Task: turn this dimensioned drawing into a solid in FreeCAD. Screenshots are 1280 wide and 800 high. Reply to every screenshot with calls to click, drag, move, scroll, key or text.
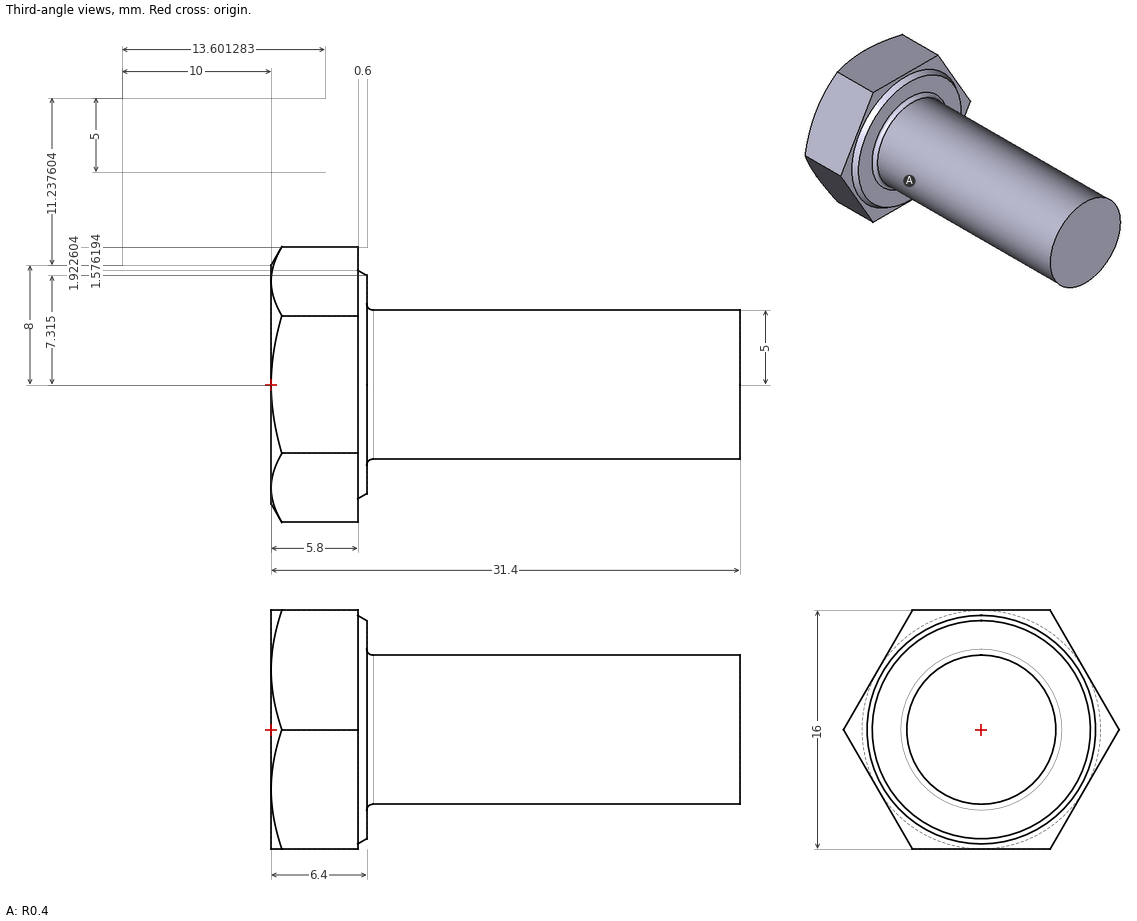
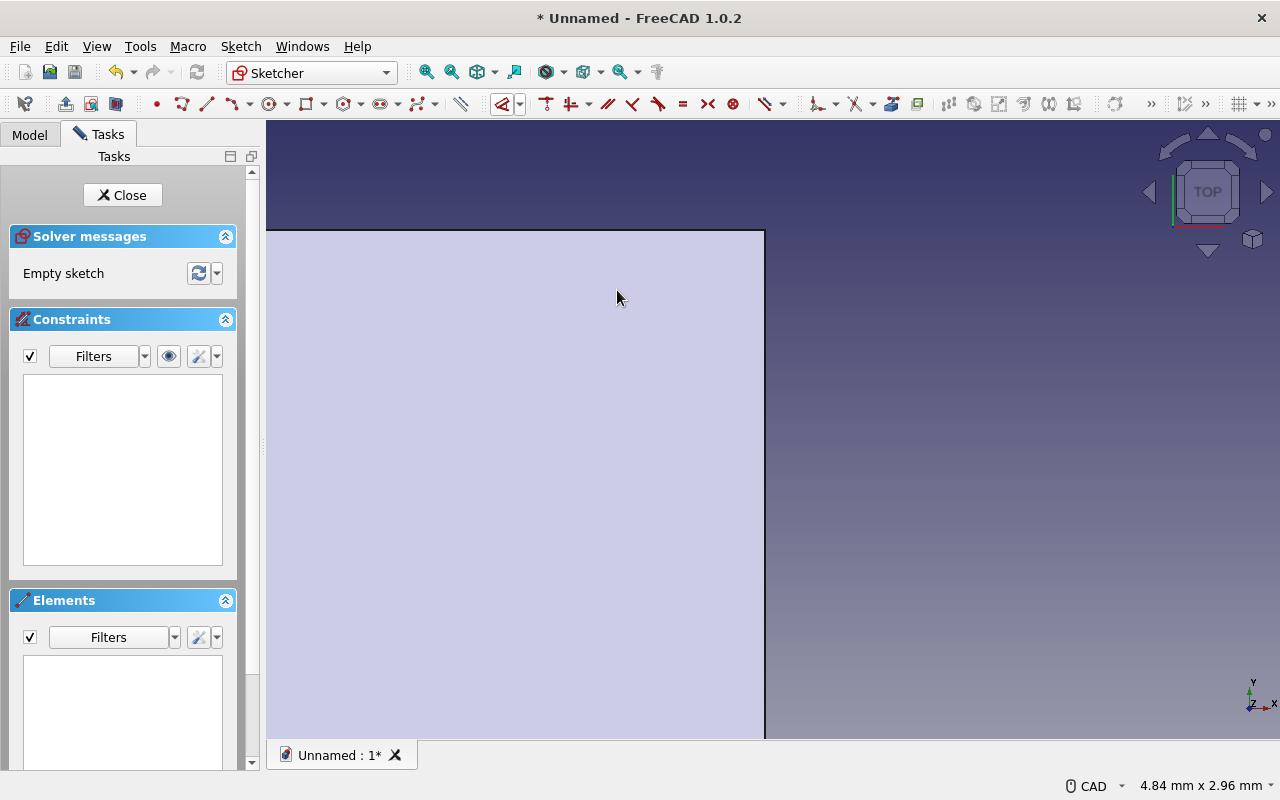
click(182, 104)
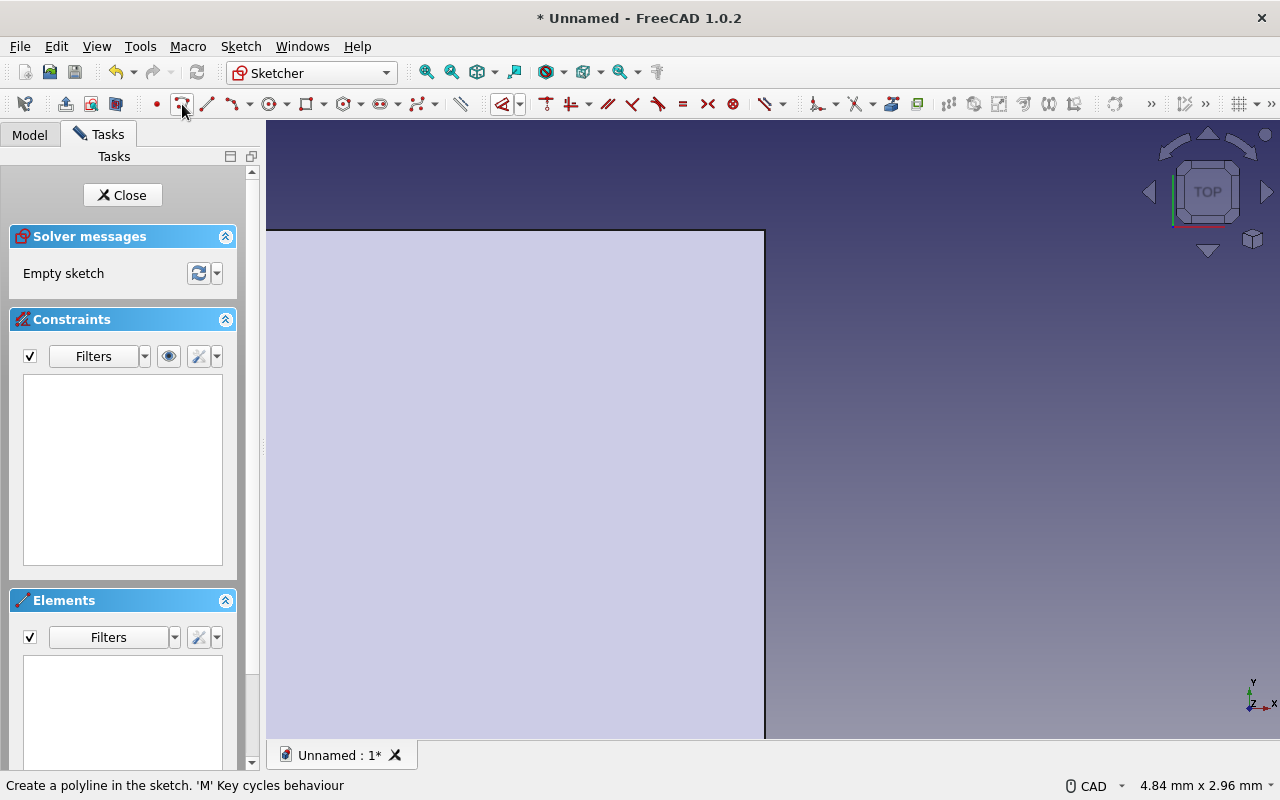
click(639, 560)
click(765, 633)
click(765, 230)
click(639, 230)
click(639, 561)
key(Escape)
key(Escape)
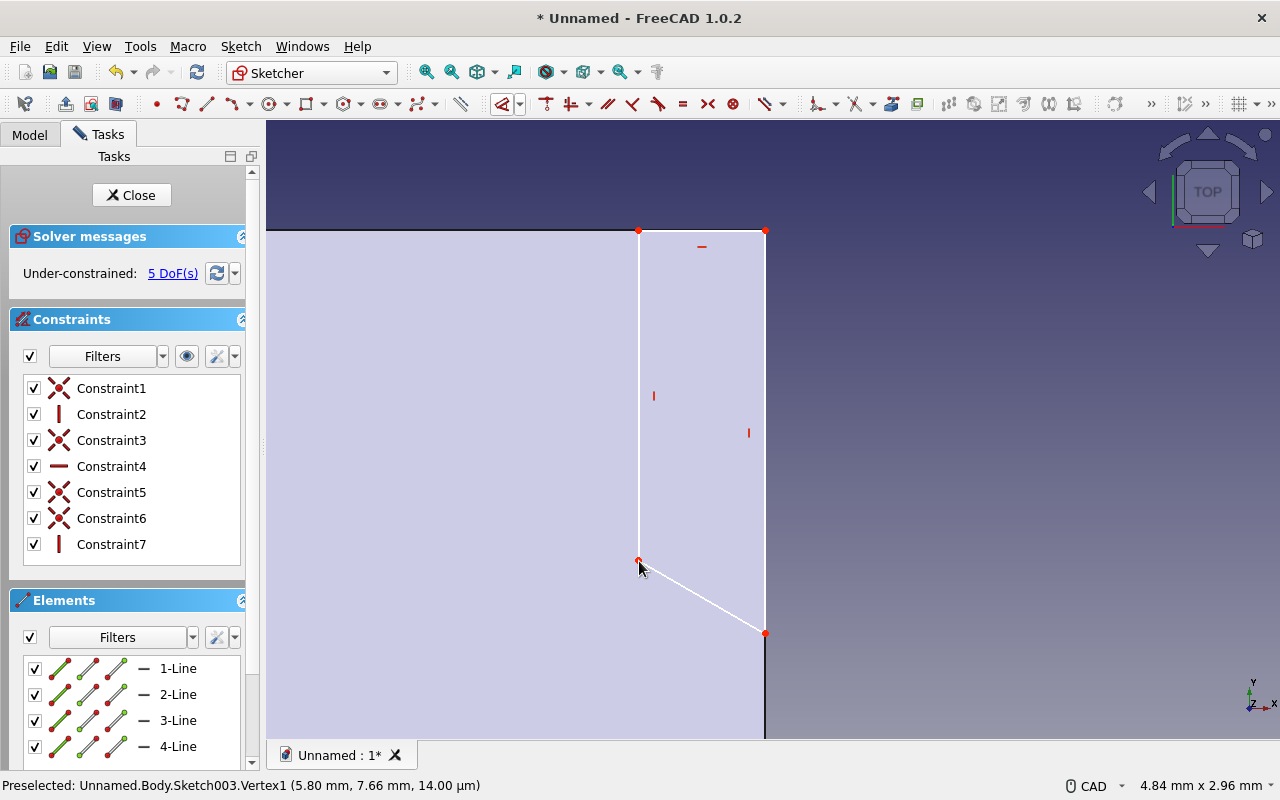
click(727, 231)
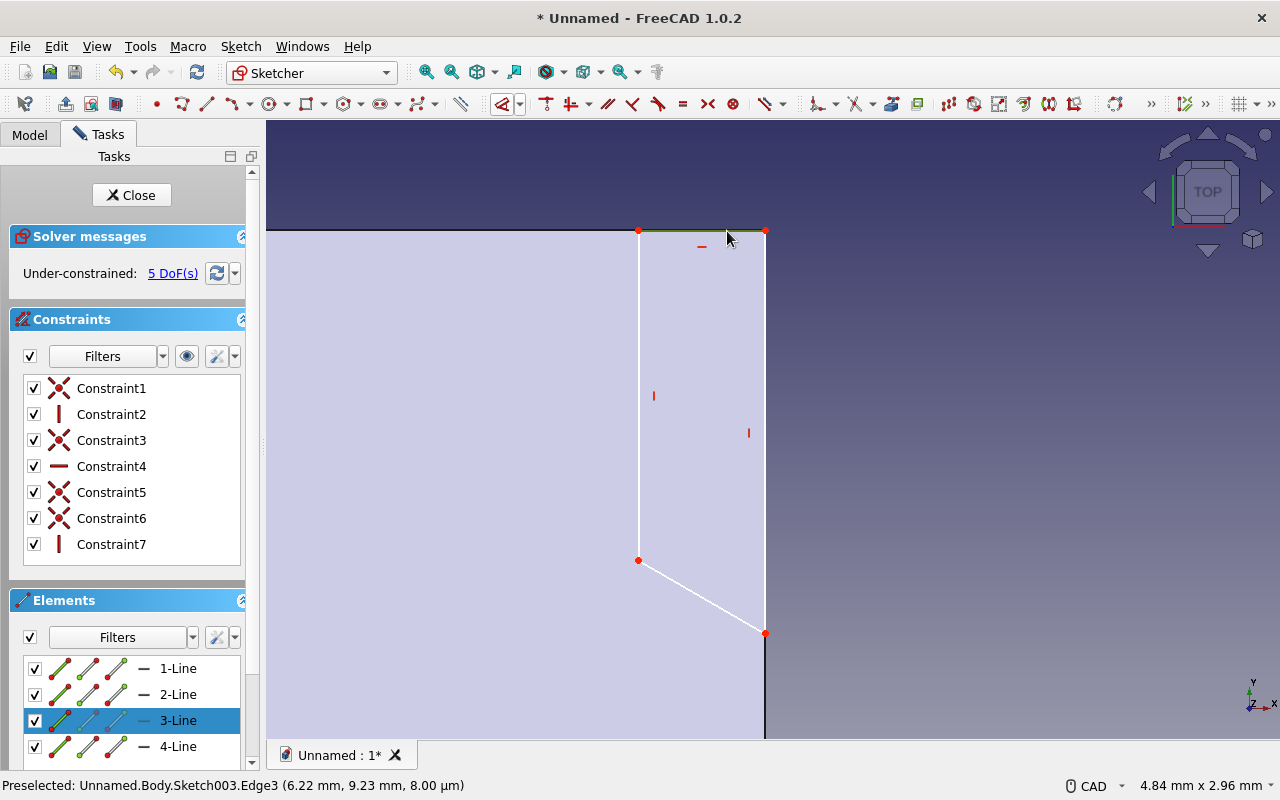
click(520, 104)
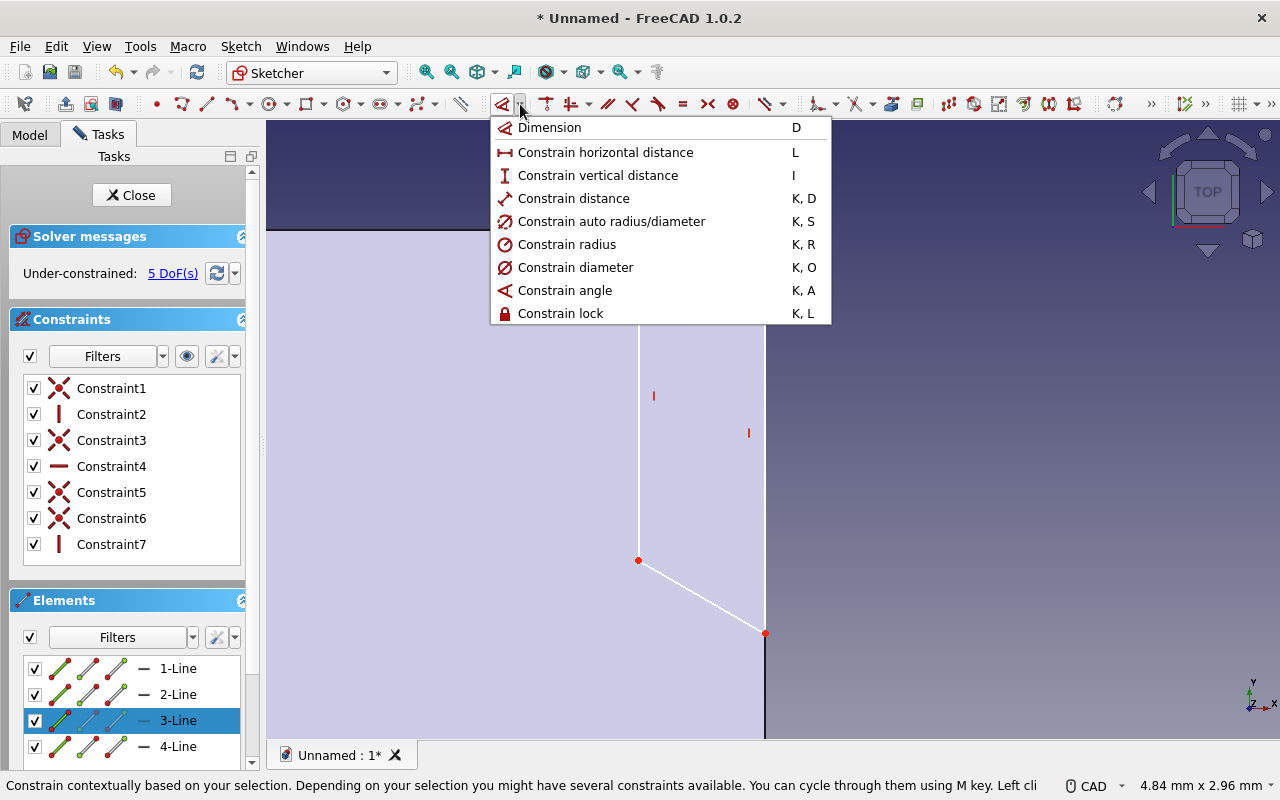
click(661, 152)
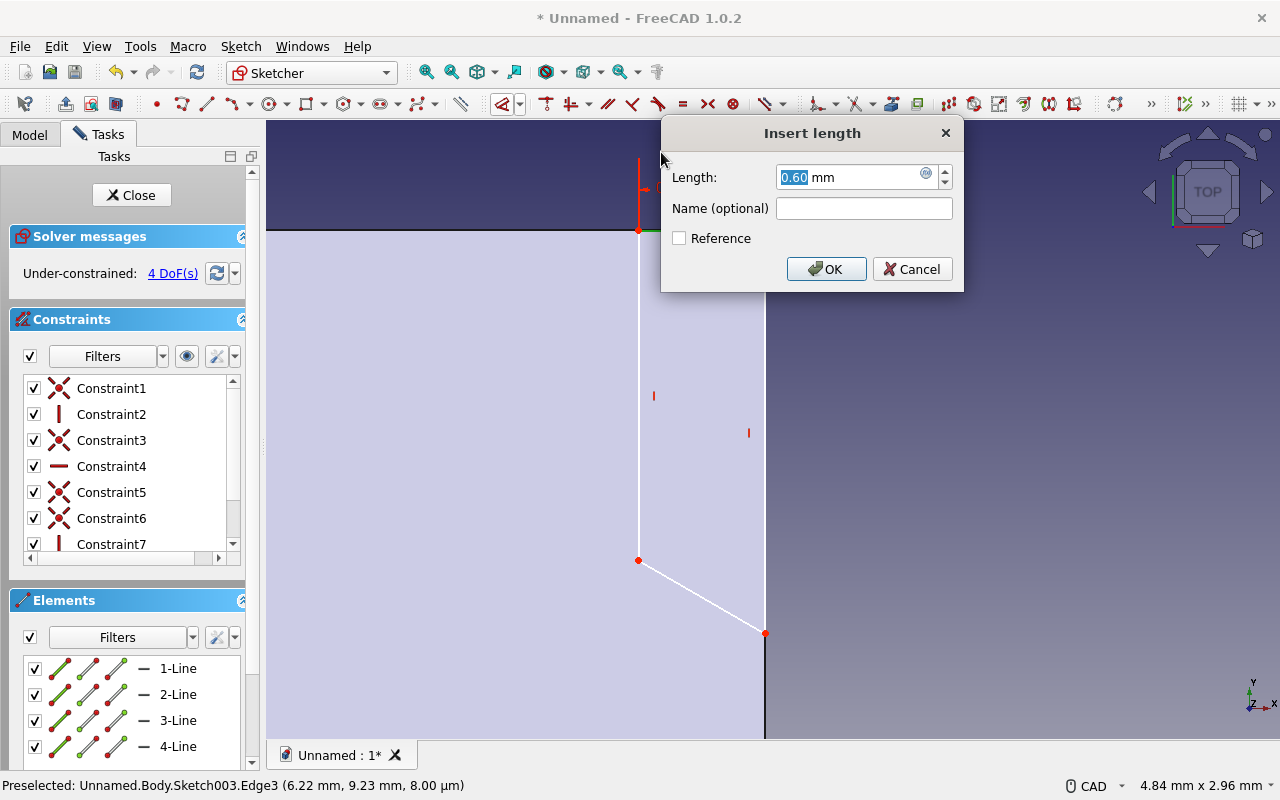
text(0.6)
key(Return)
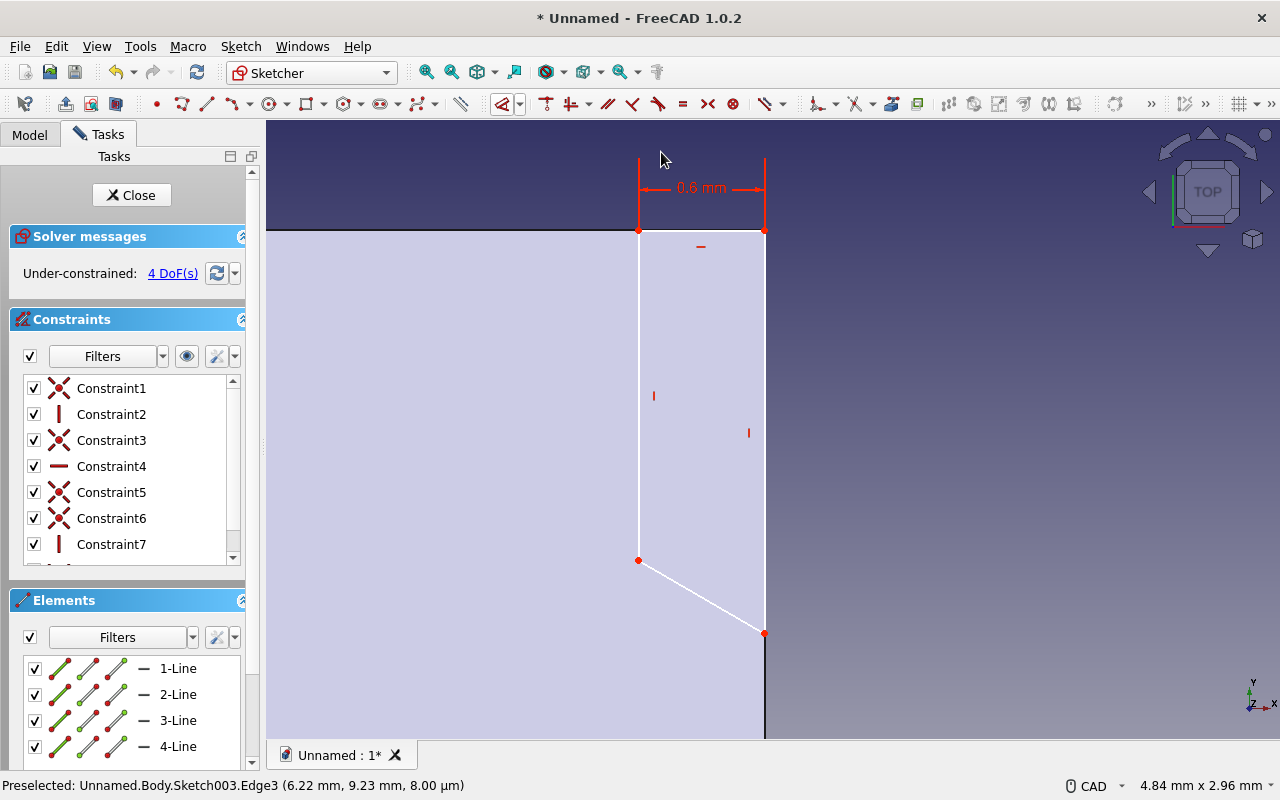
click(639, 561)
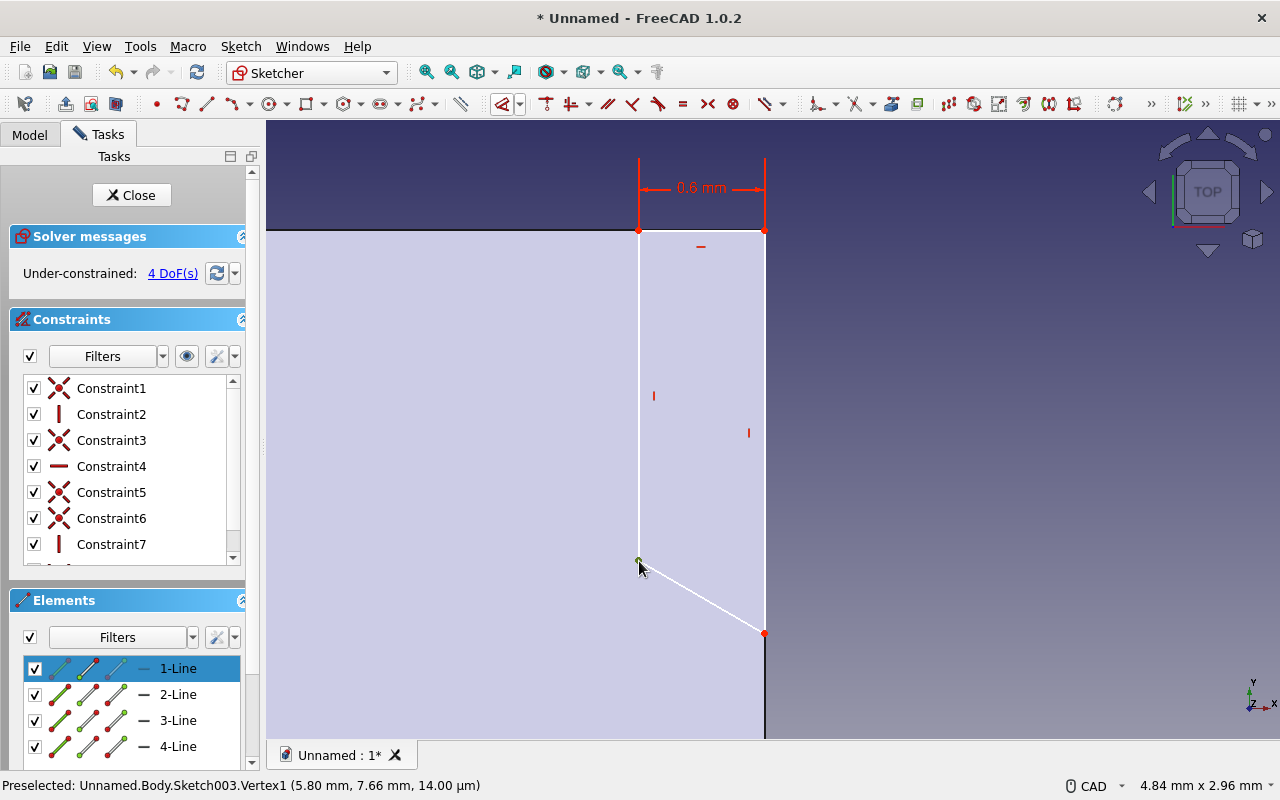
key(l)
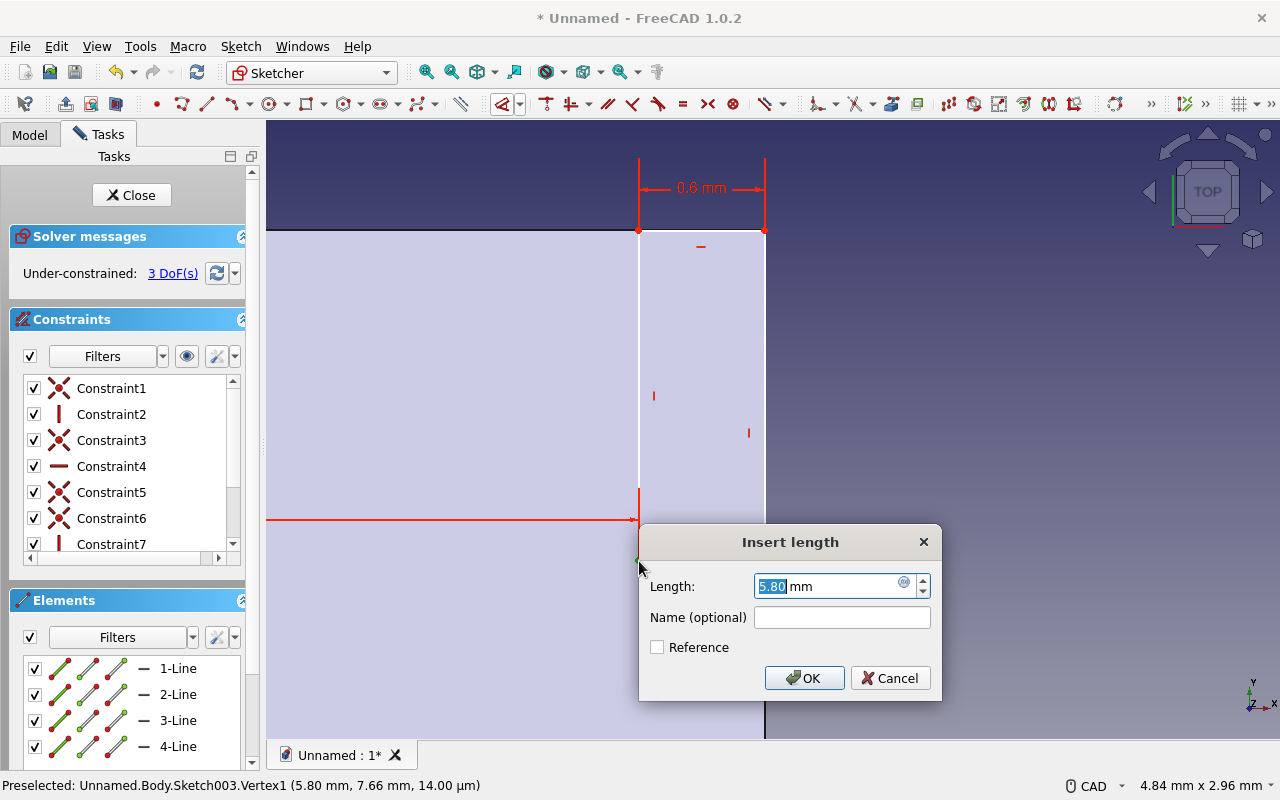
text(5.8)
key(Return)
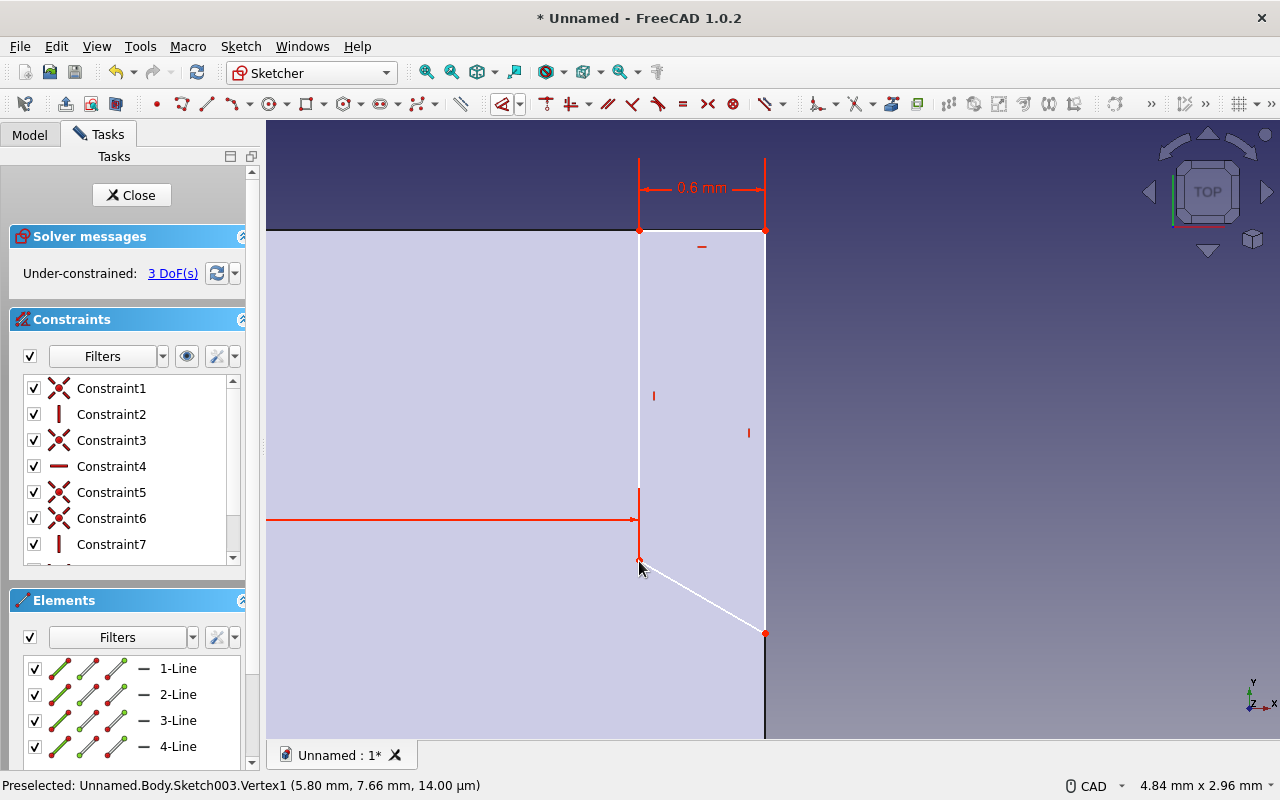
click(765, 634)